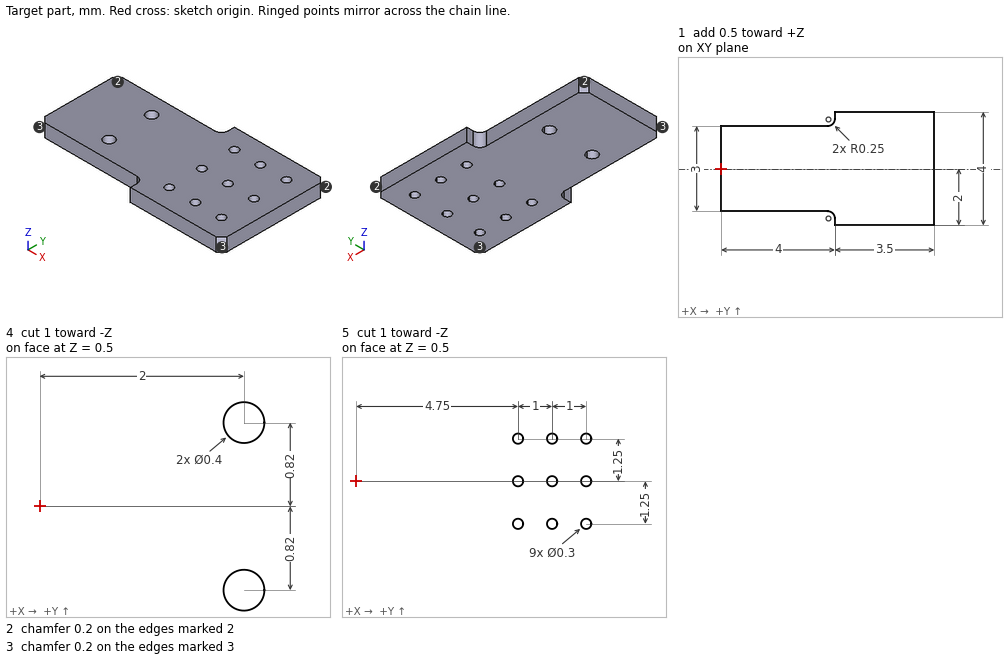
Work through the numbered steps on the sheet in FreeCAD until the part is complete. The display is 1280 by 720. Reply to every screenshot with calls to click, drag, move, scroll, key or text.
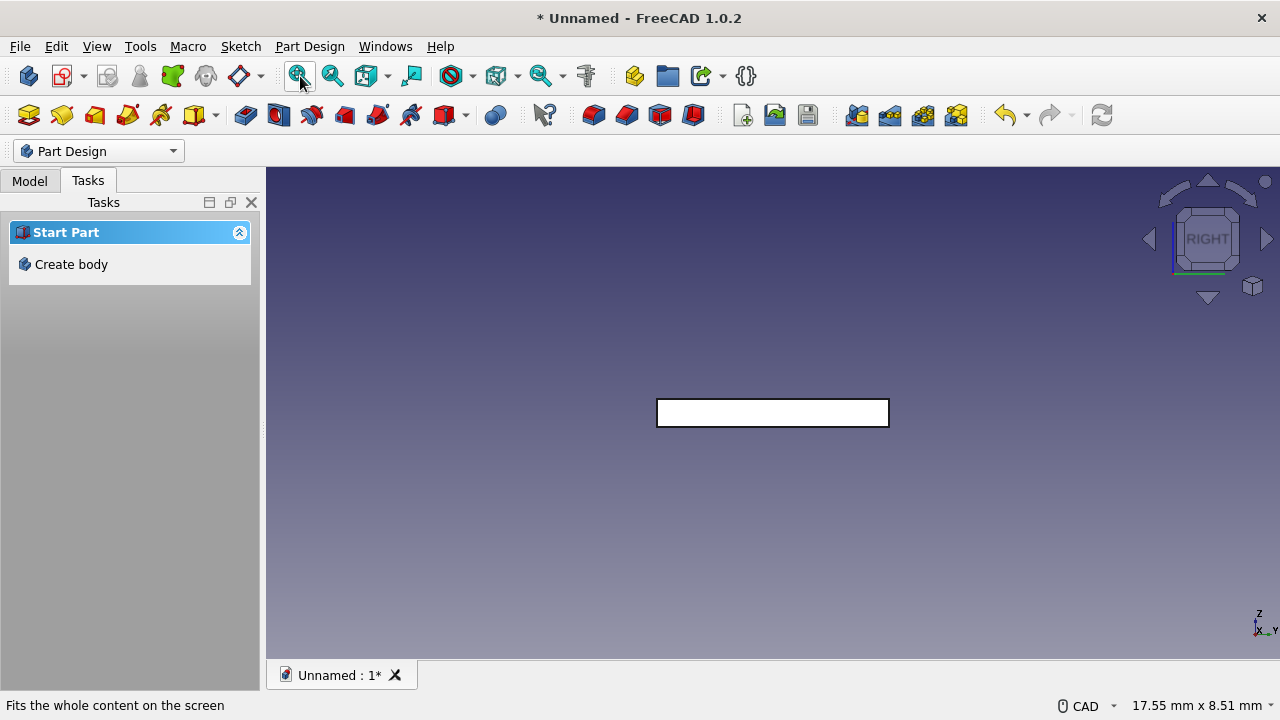
key(v)
key(f)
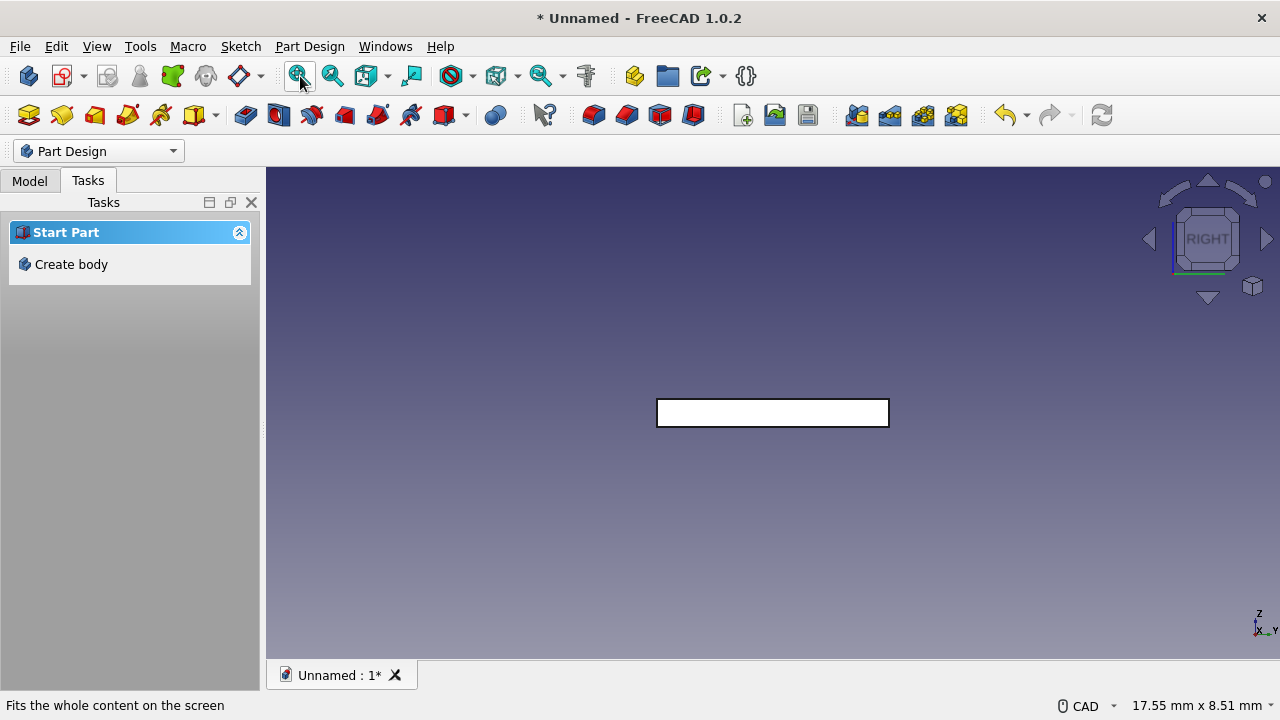
click(889, 412)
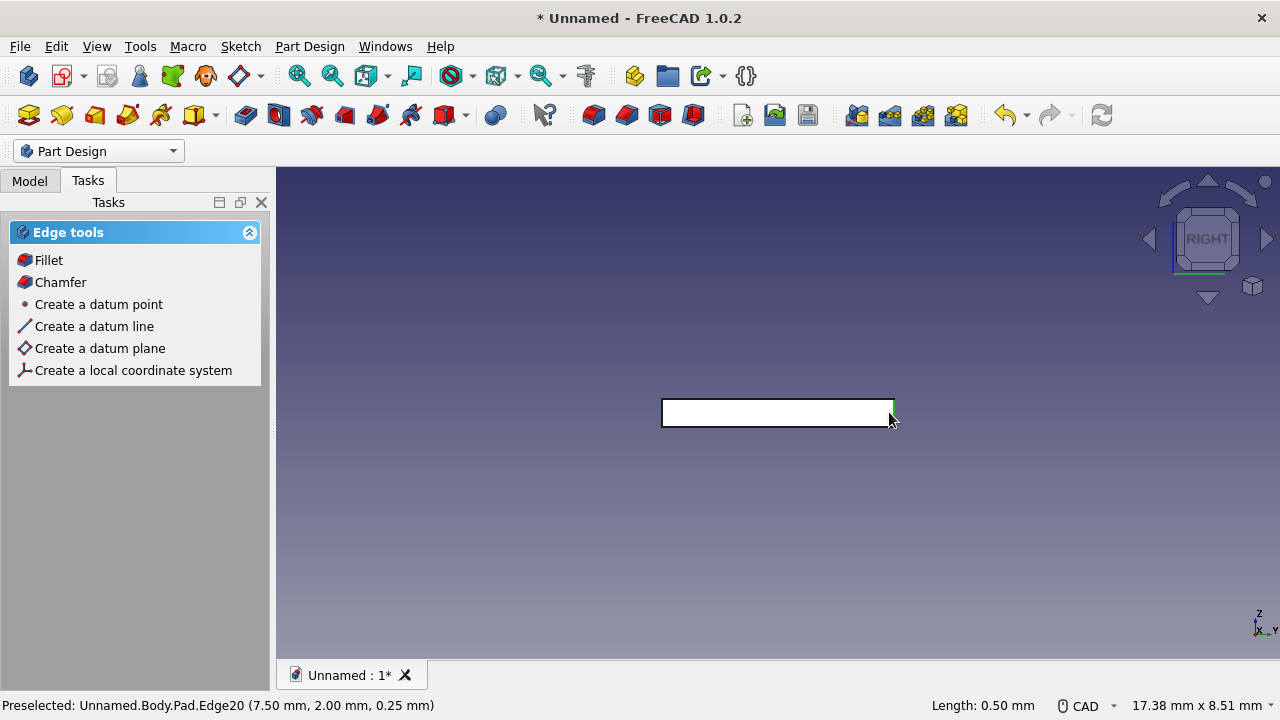
key(5)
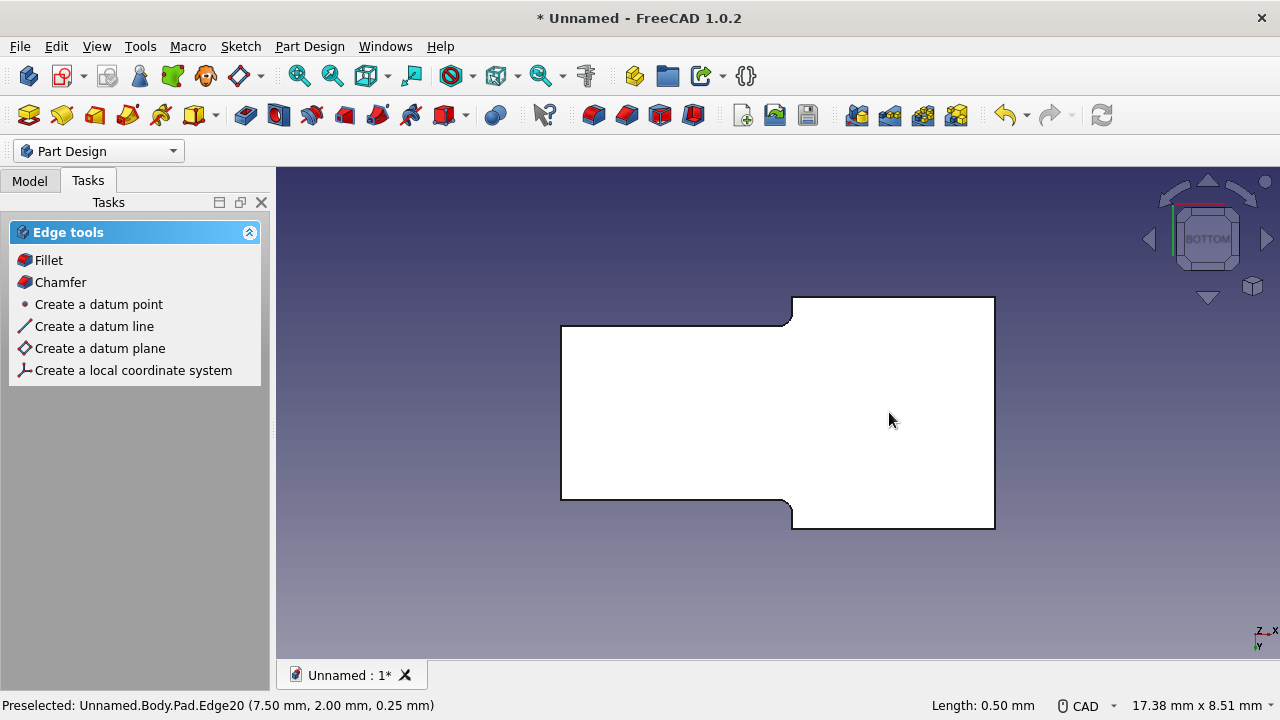
key(4)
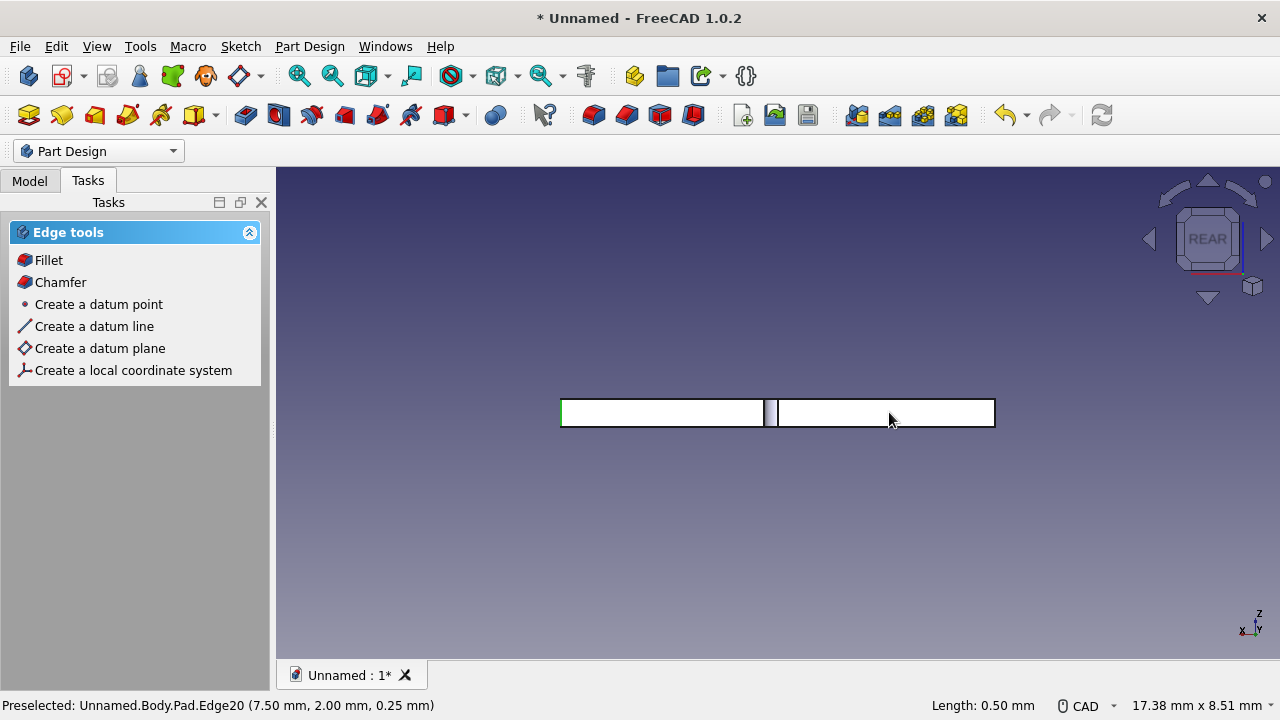
key(v)
key(f)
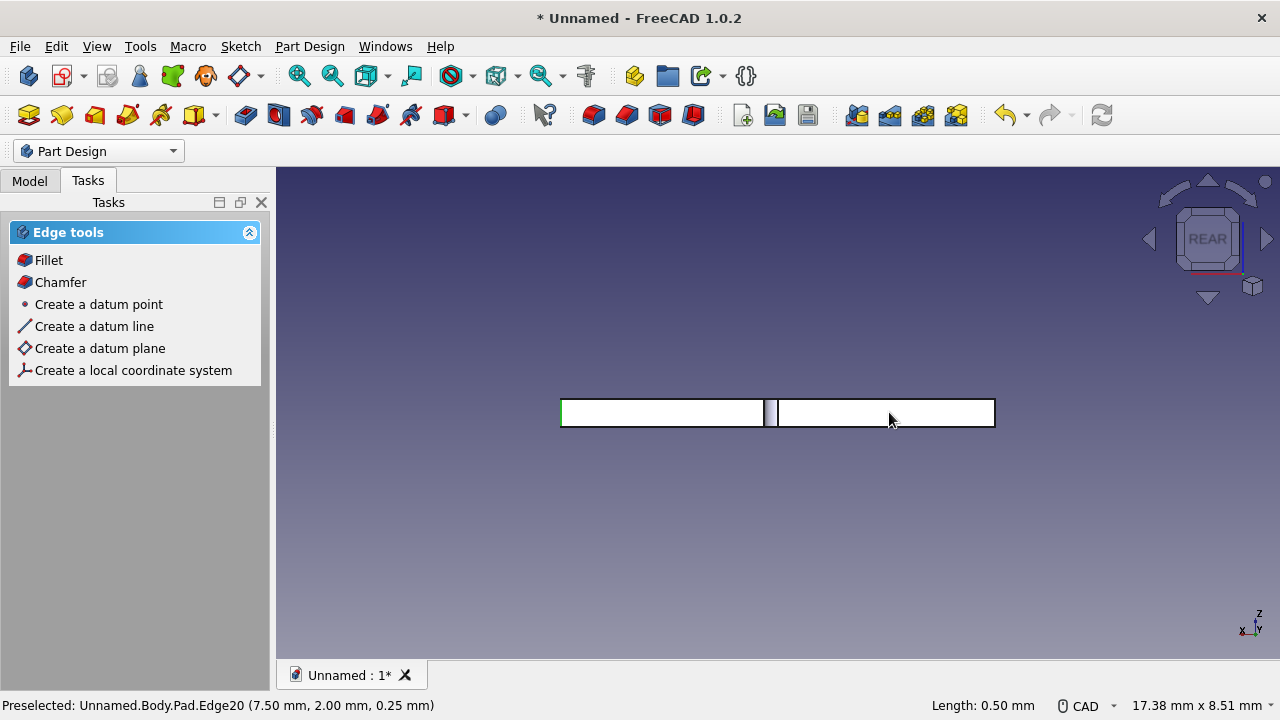
click(995, 412, ctrl)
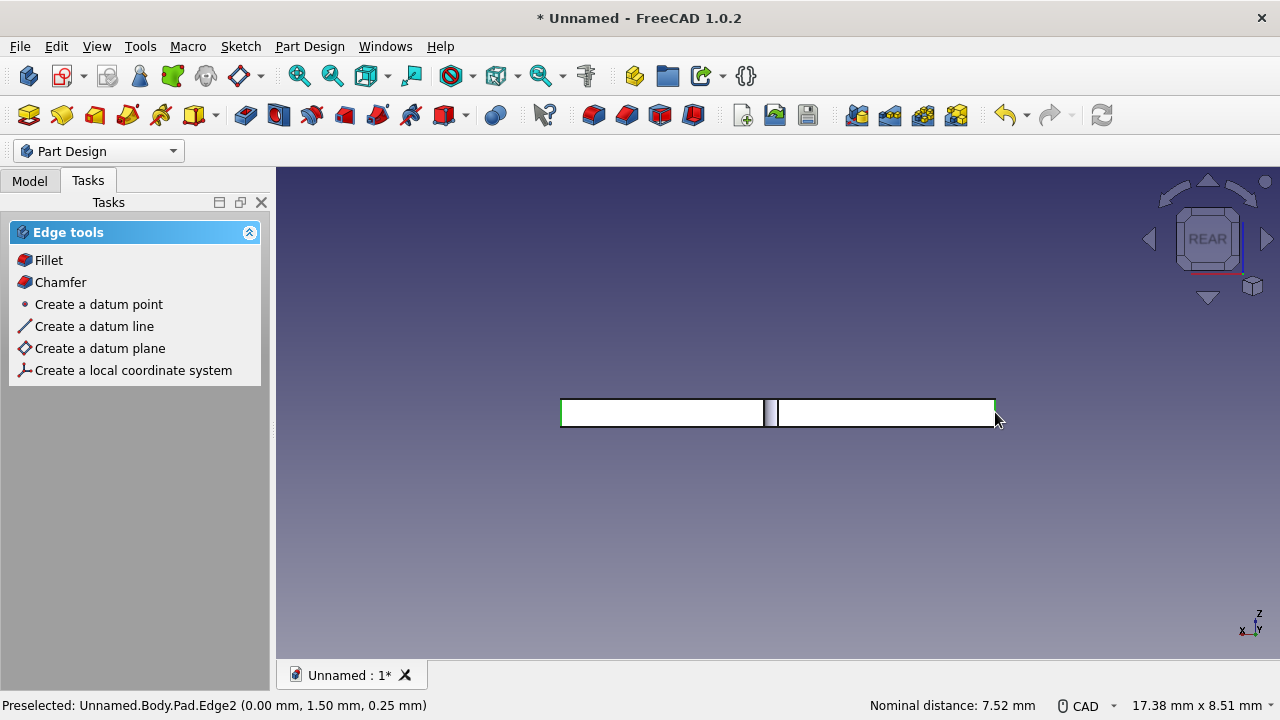
click(627, 116)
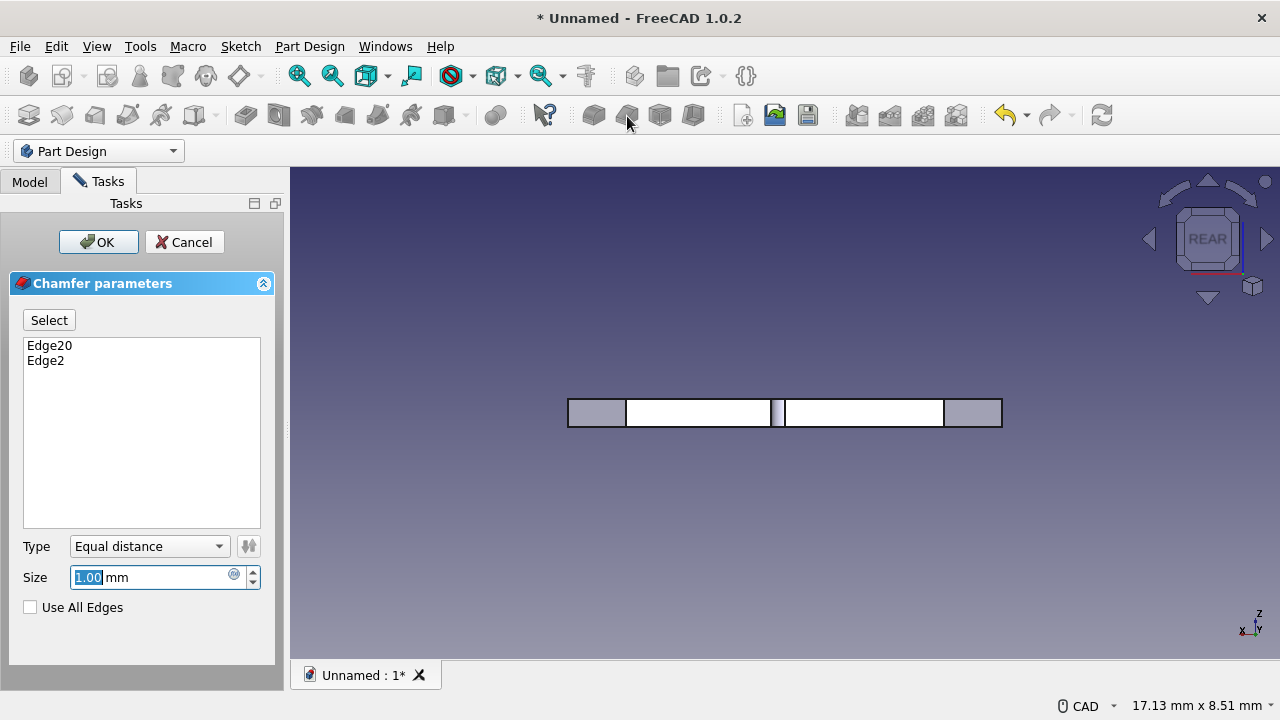
text(0.2)
key(Tab)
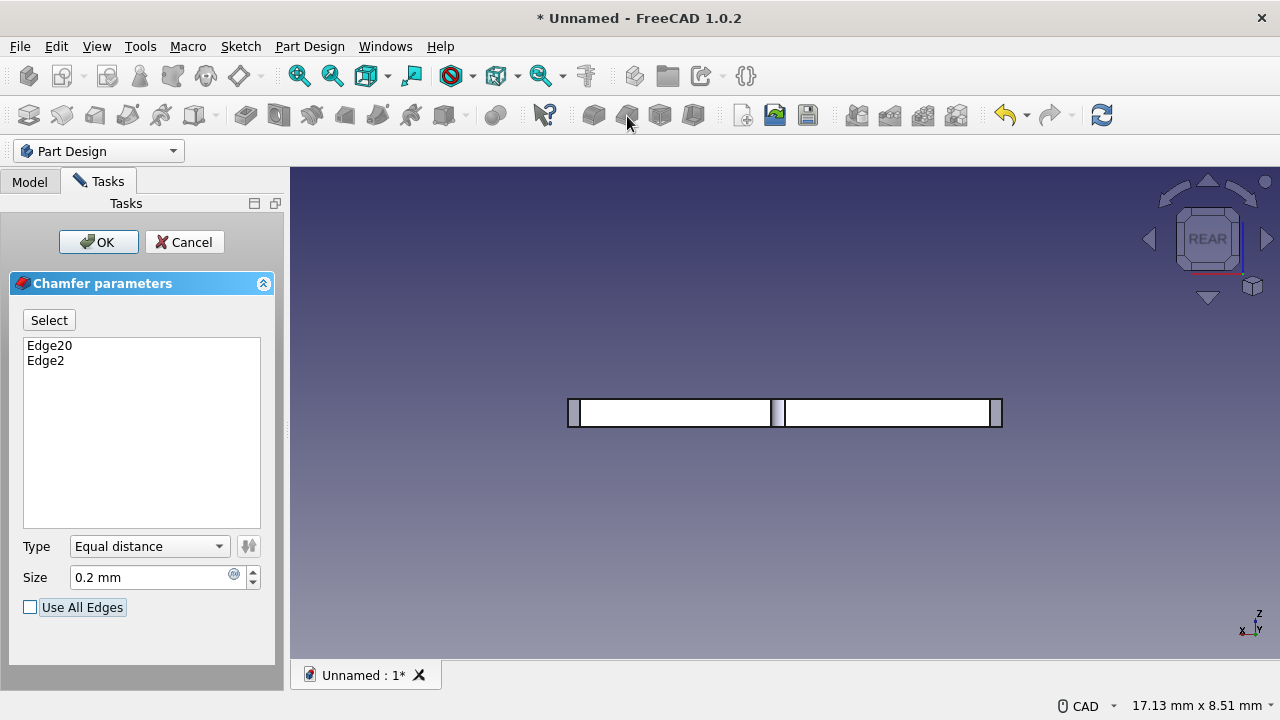
click(99, 242)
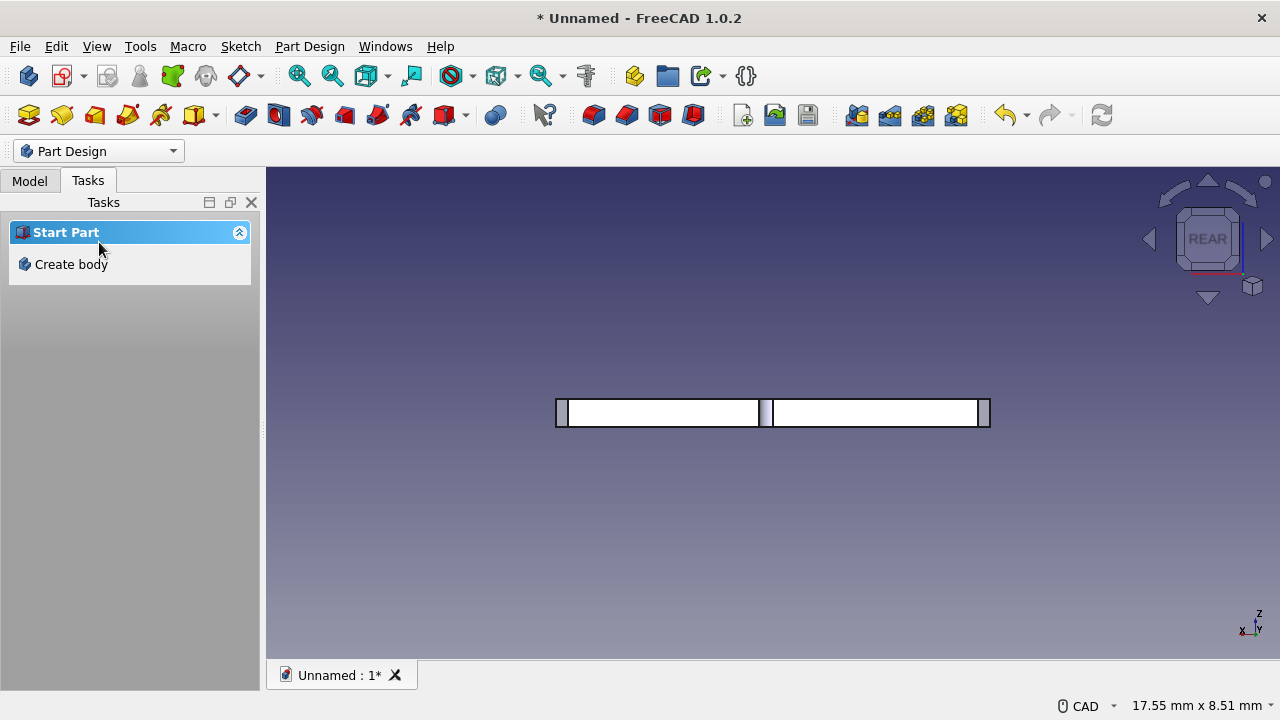
click(300, 76)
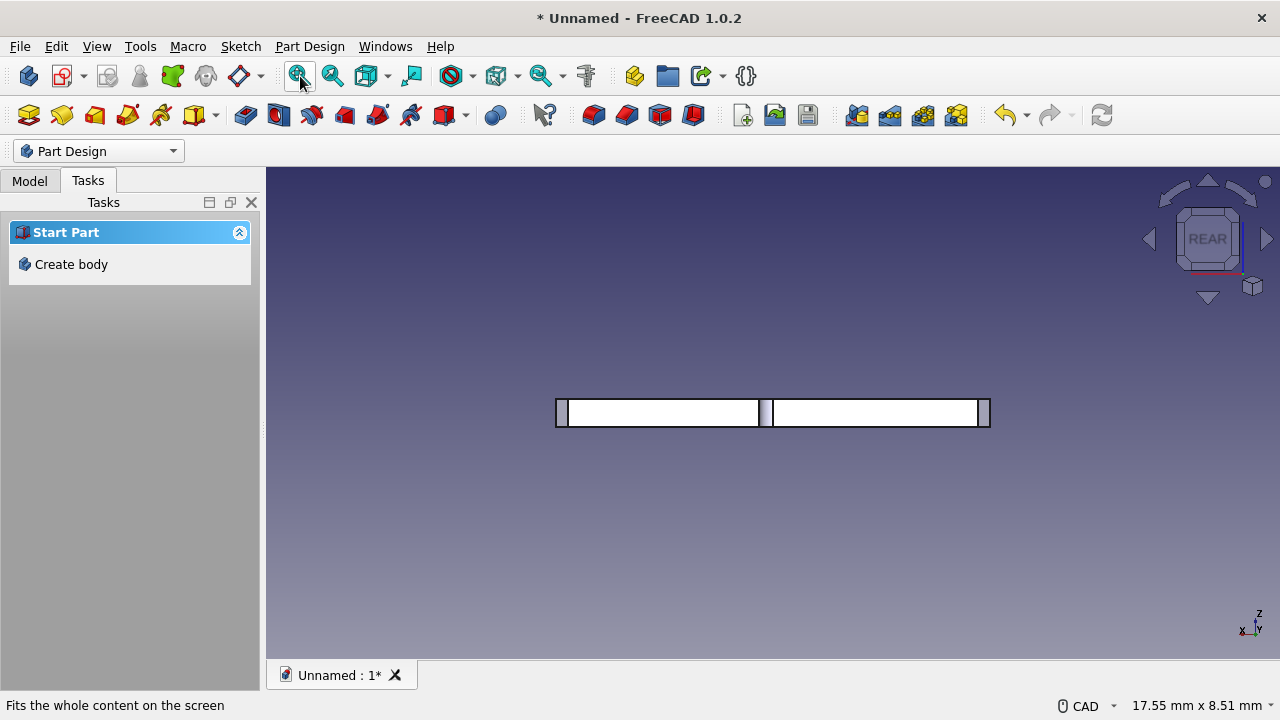
key(0)